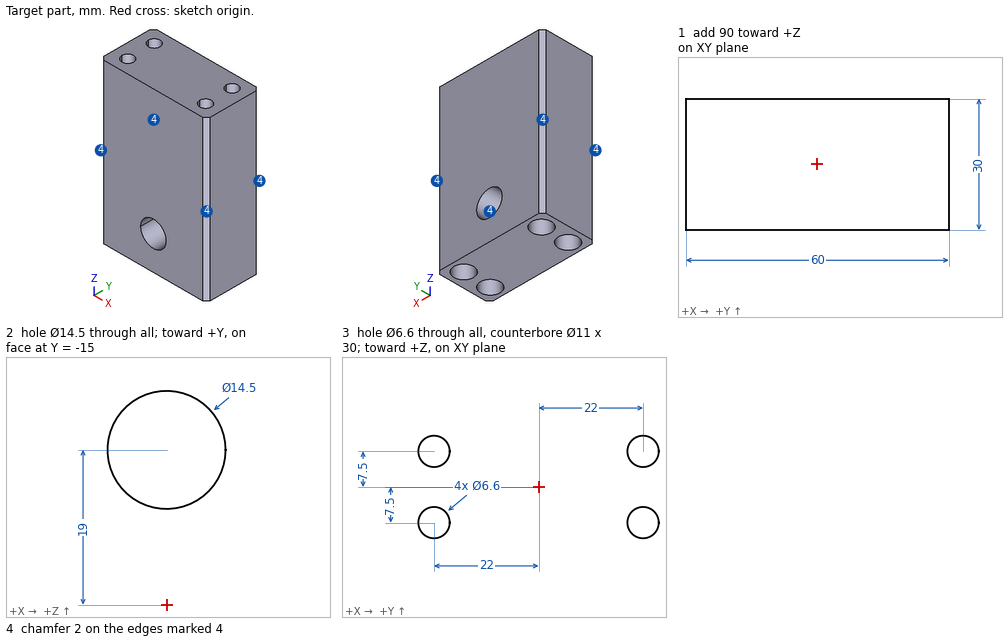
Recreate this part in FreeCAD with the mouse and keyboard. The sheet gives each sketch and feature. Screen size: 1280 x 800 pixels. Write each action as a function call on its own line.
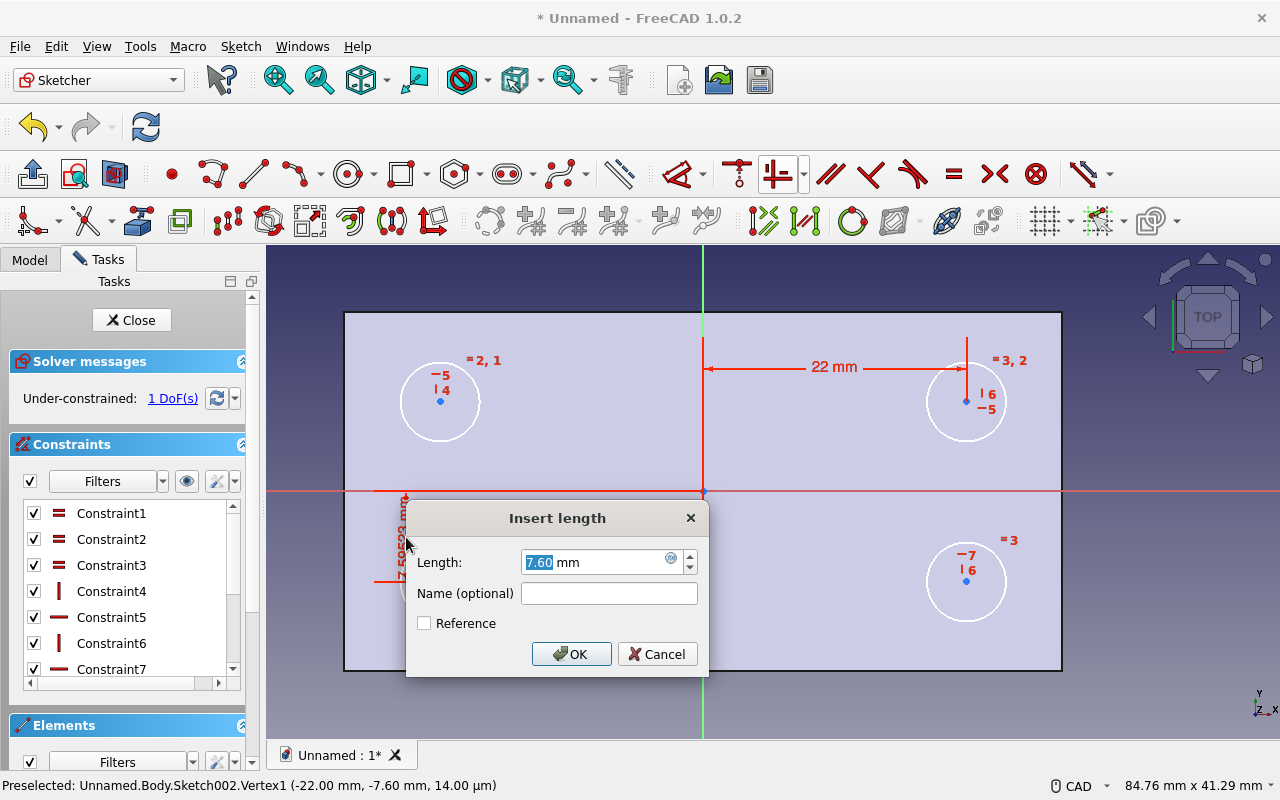
text(7.5)
key(Return)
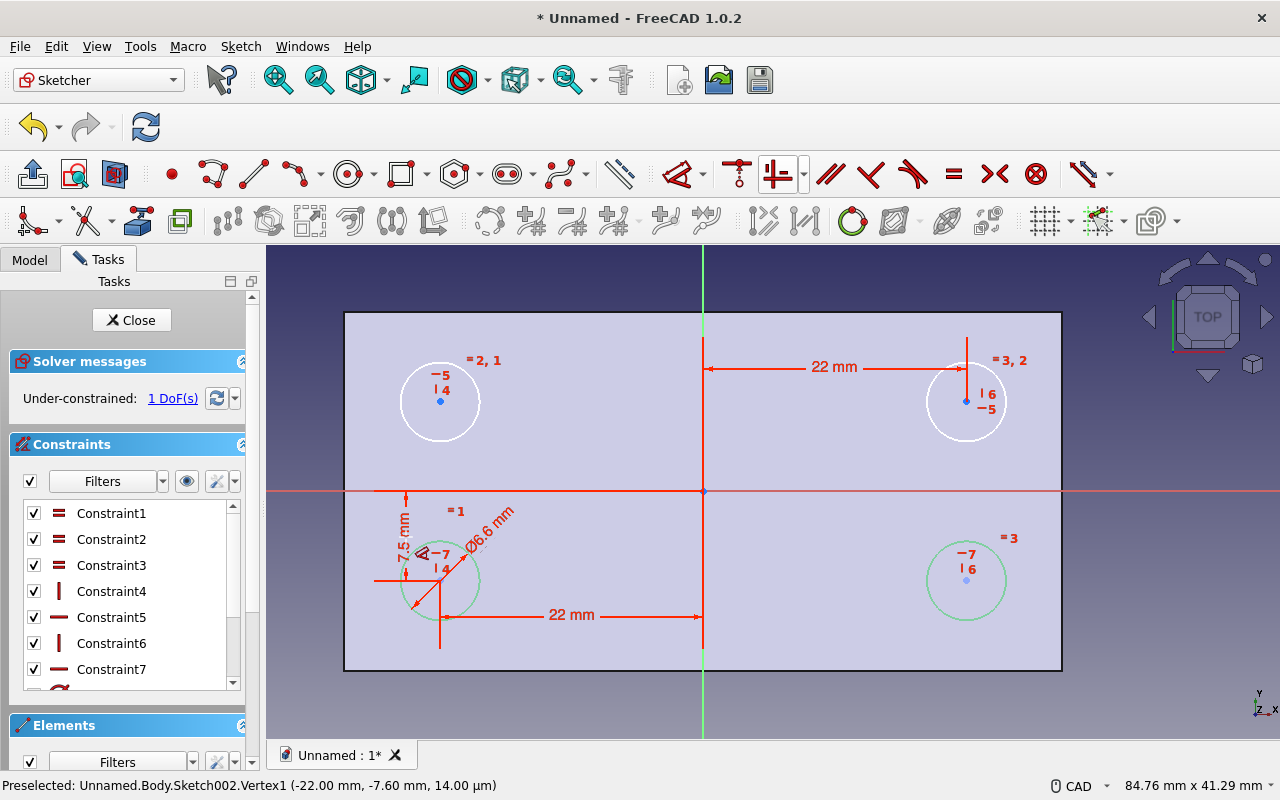
click(440, 402)
click(406, 447)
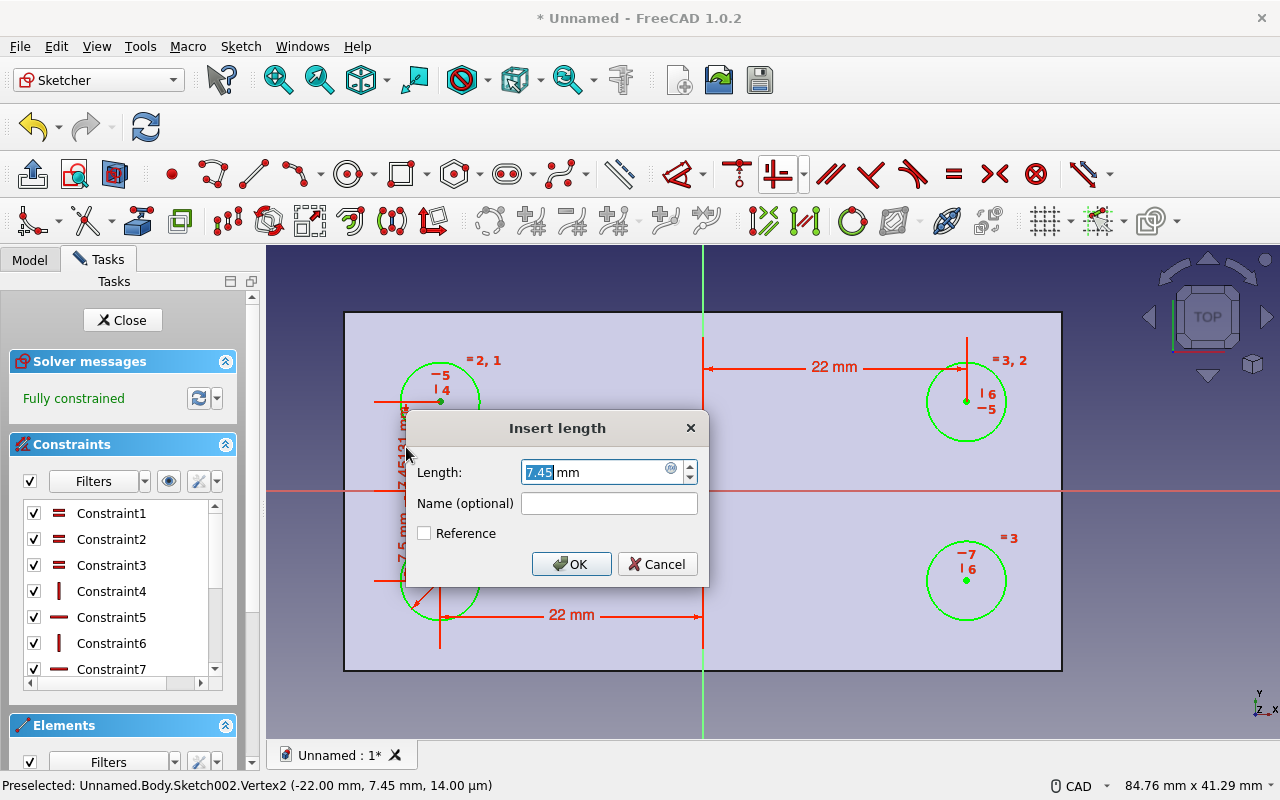
text(7.5)
key(Return)
key(Escape)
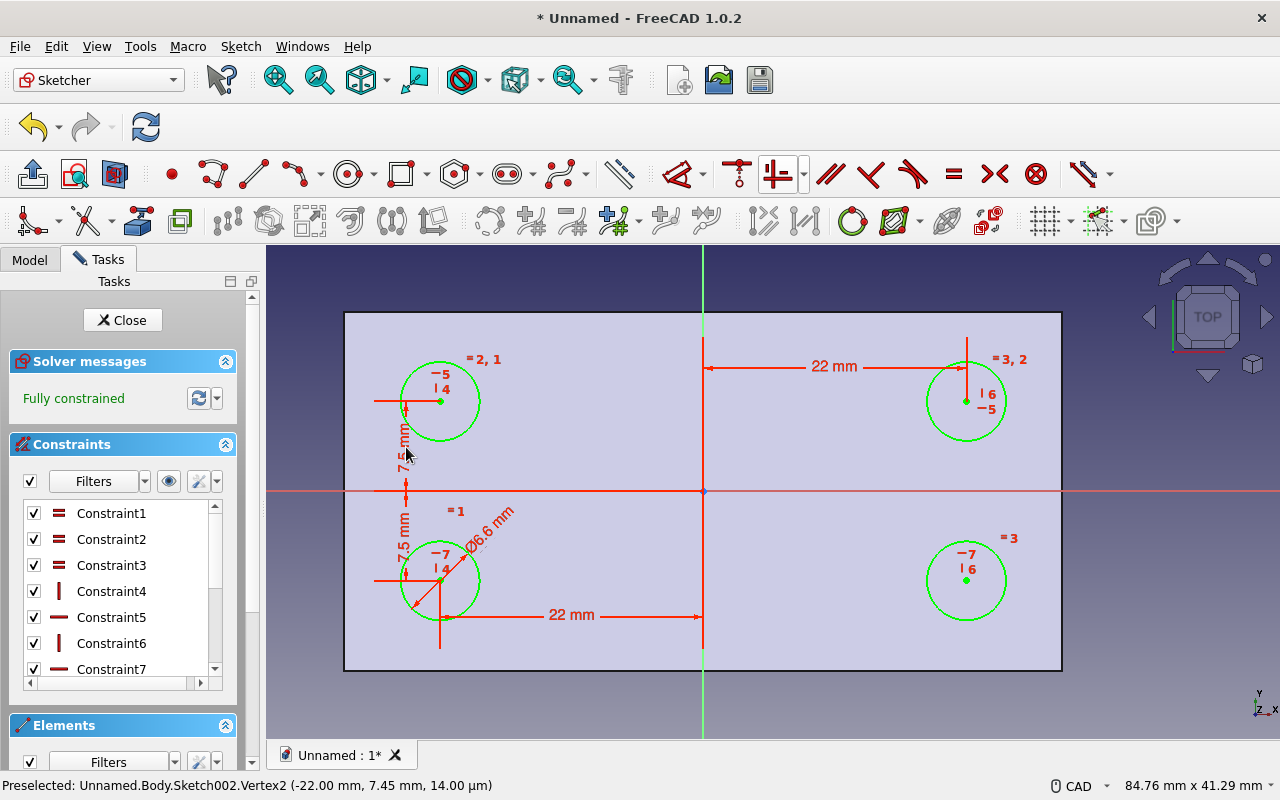
click(123, 320)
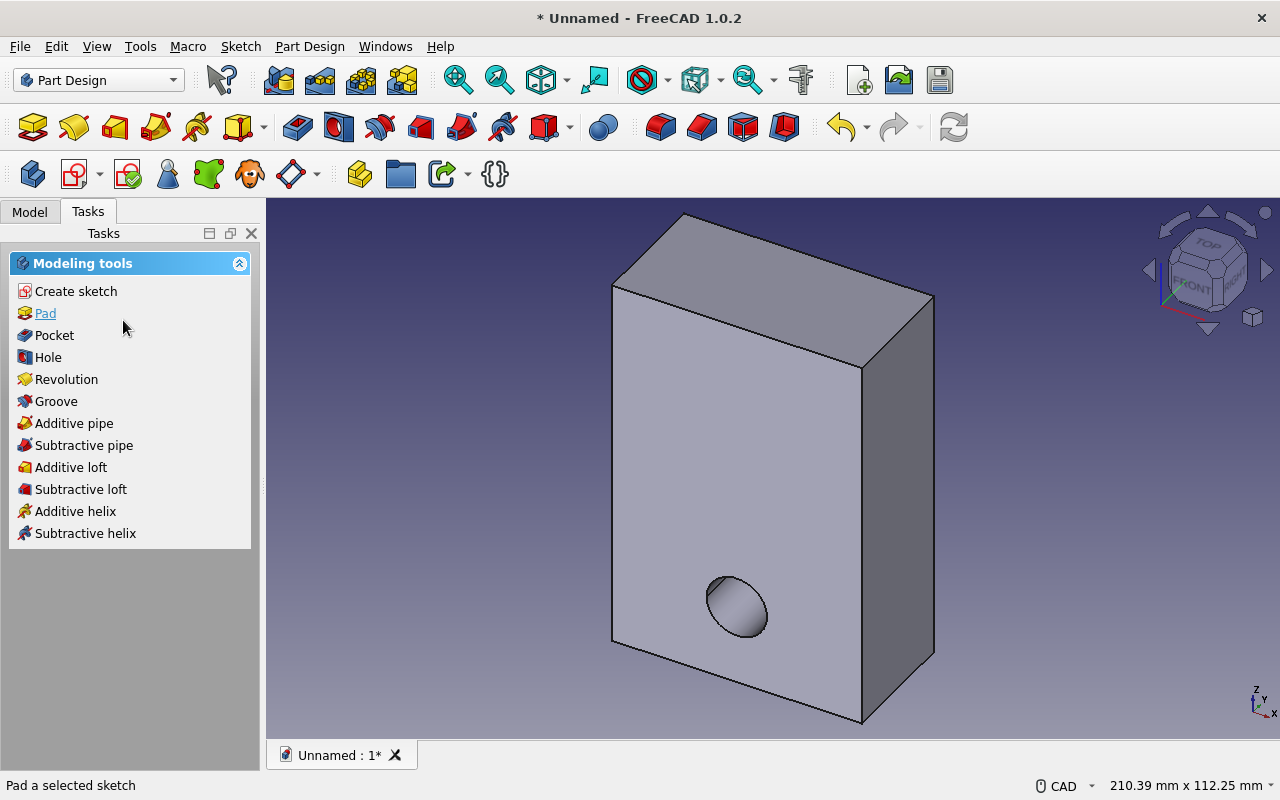
click(339, 128)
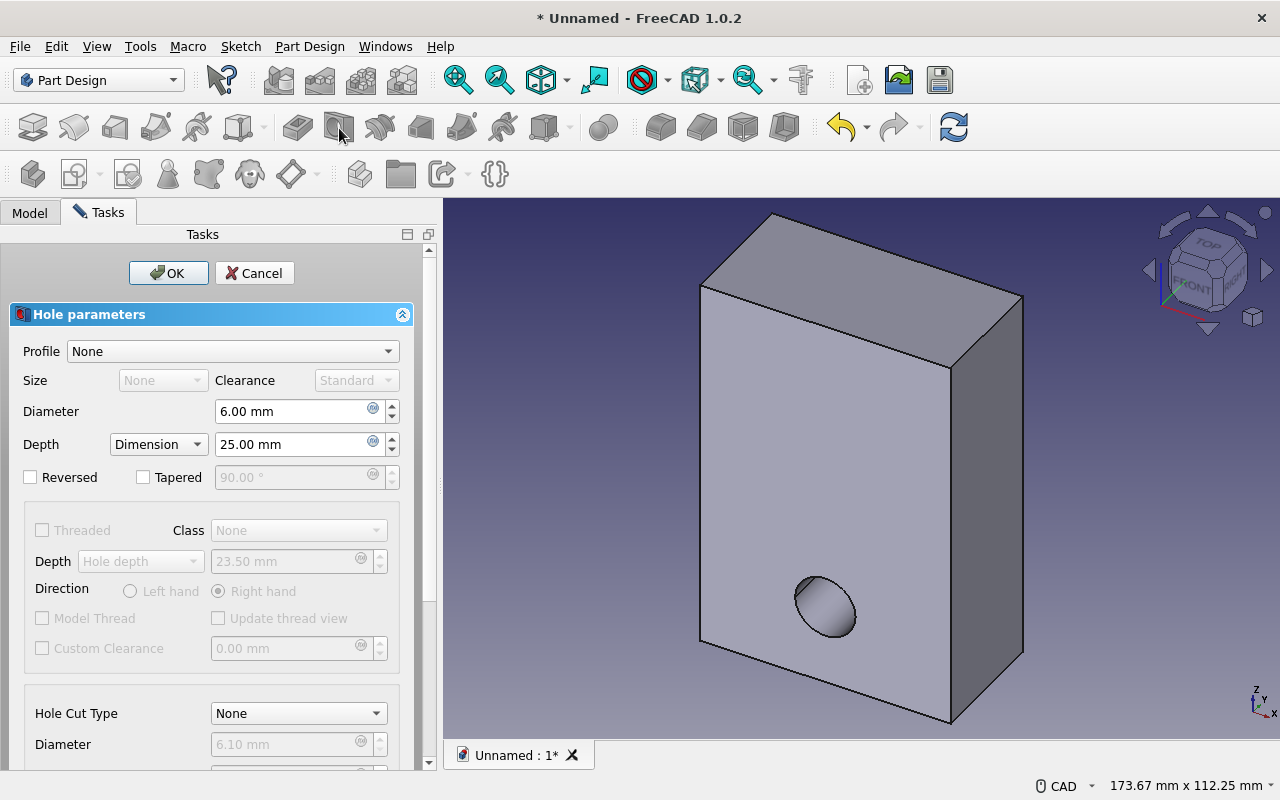
triple_click(300, 412)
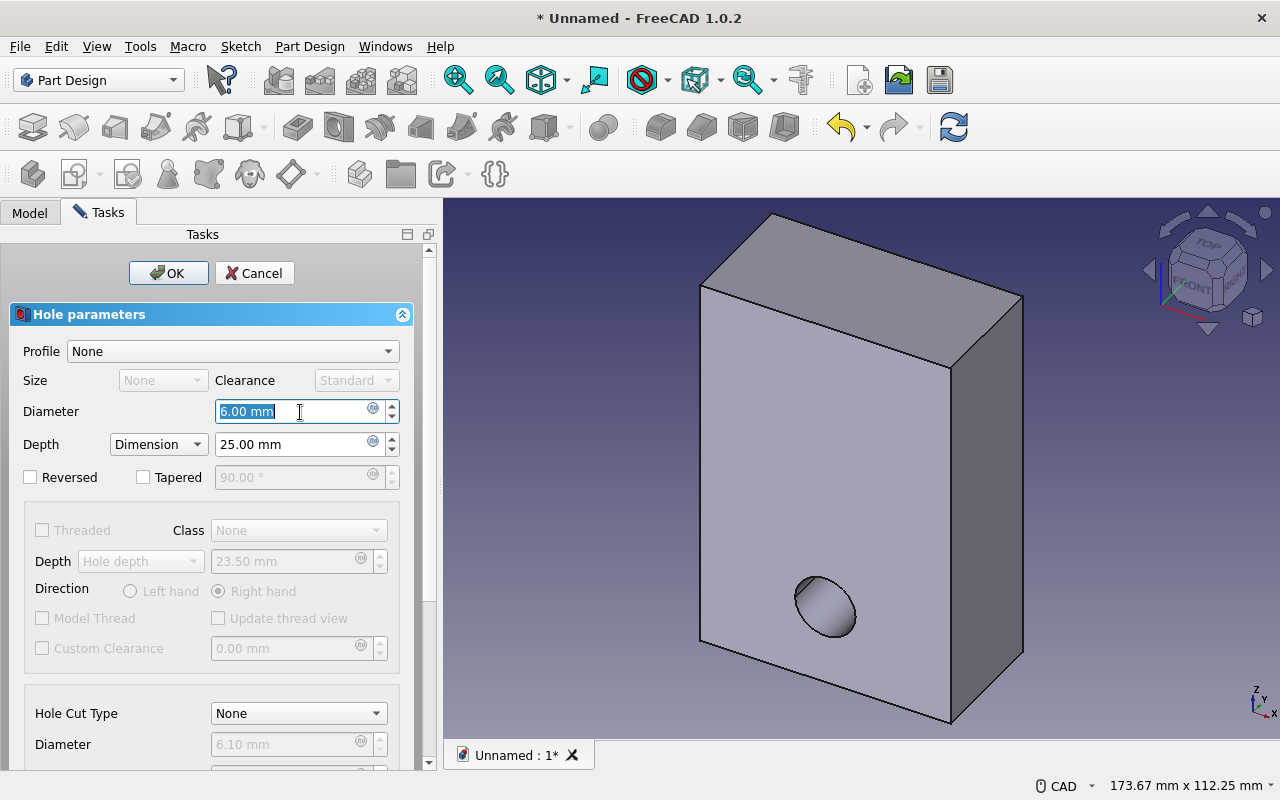
text(6.6)
key(Tab)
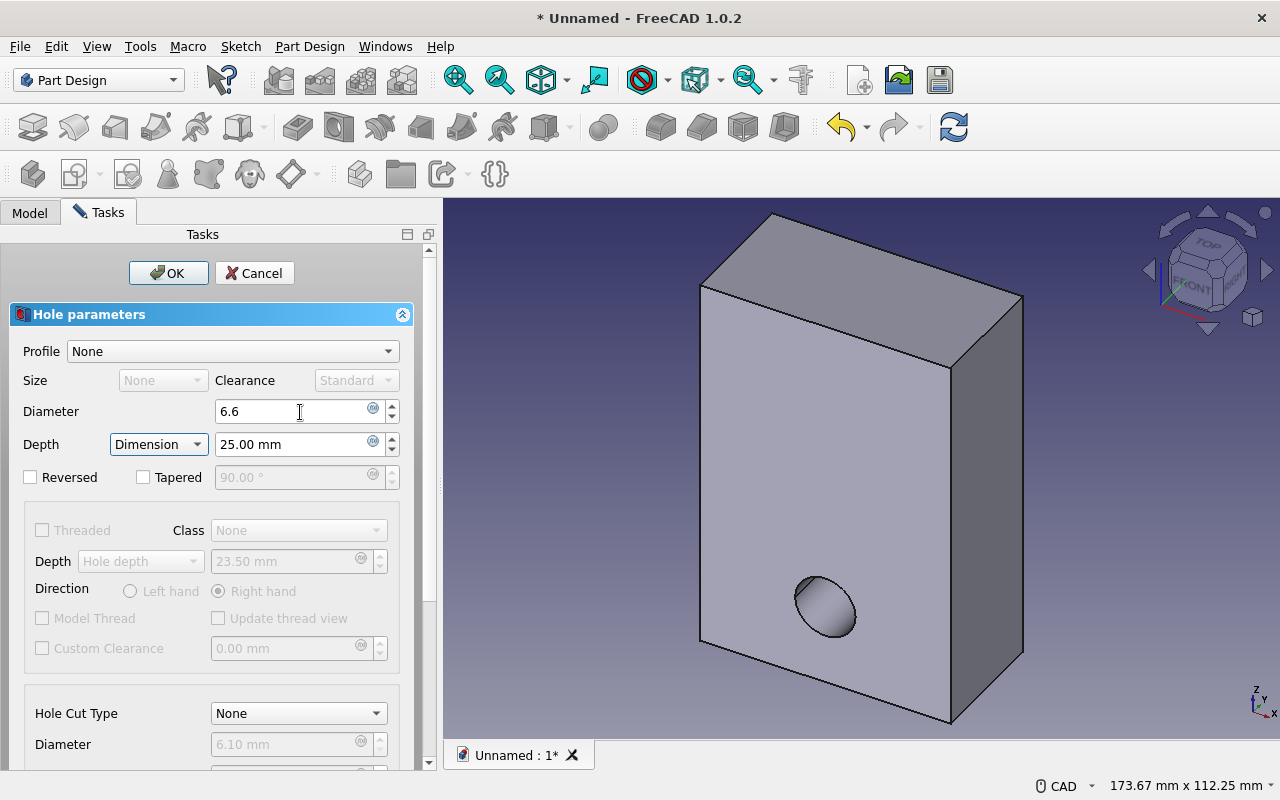
click(160, 444)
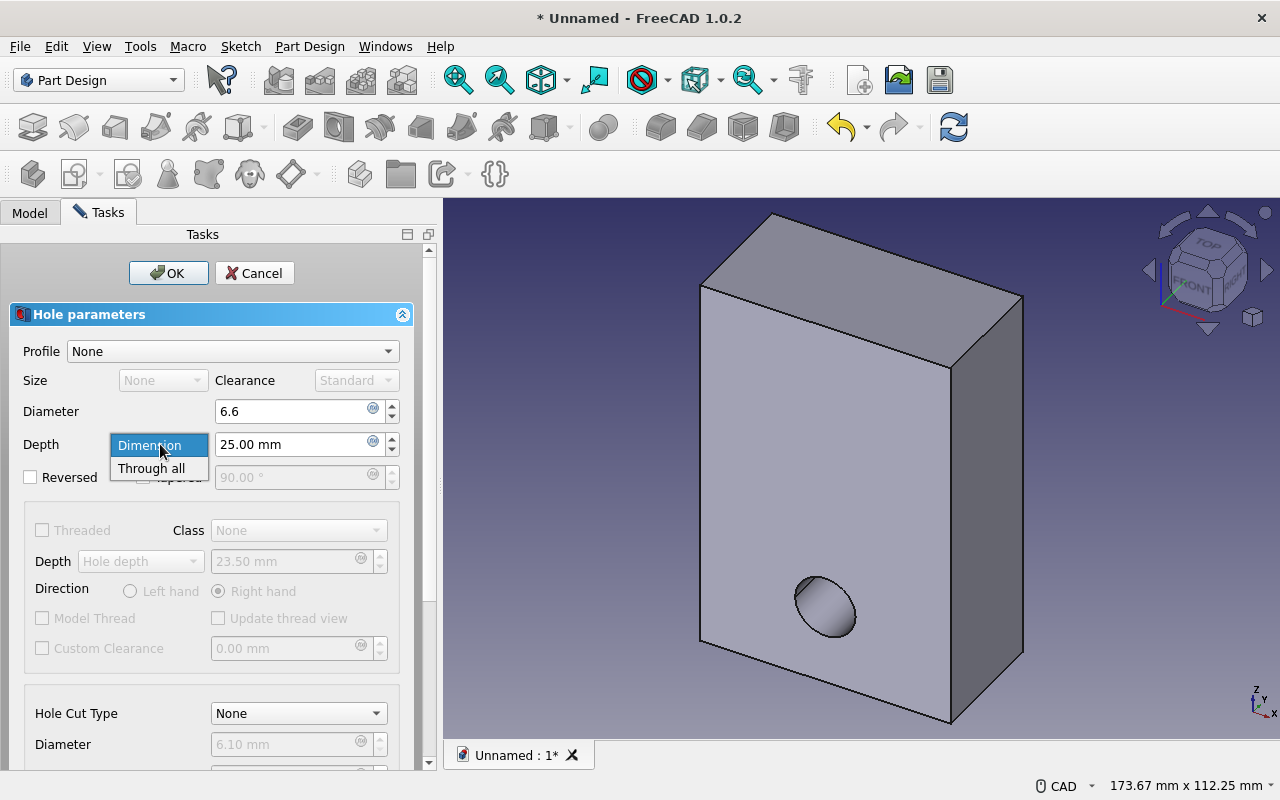
click(158, 468)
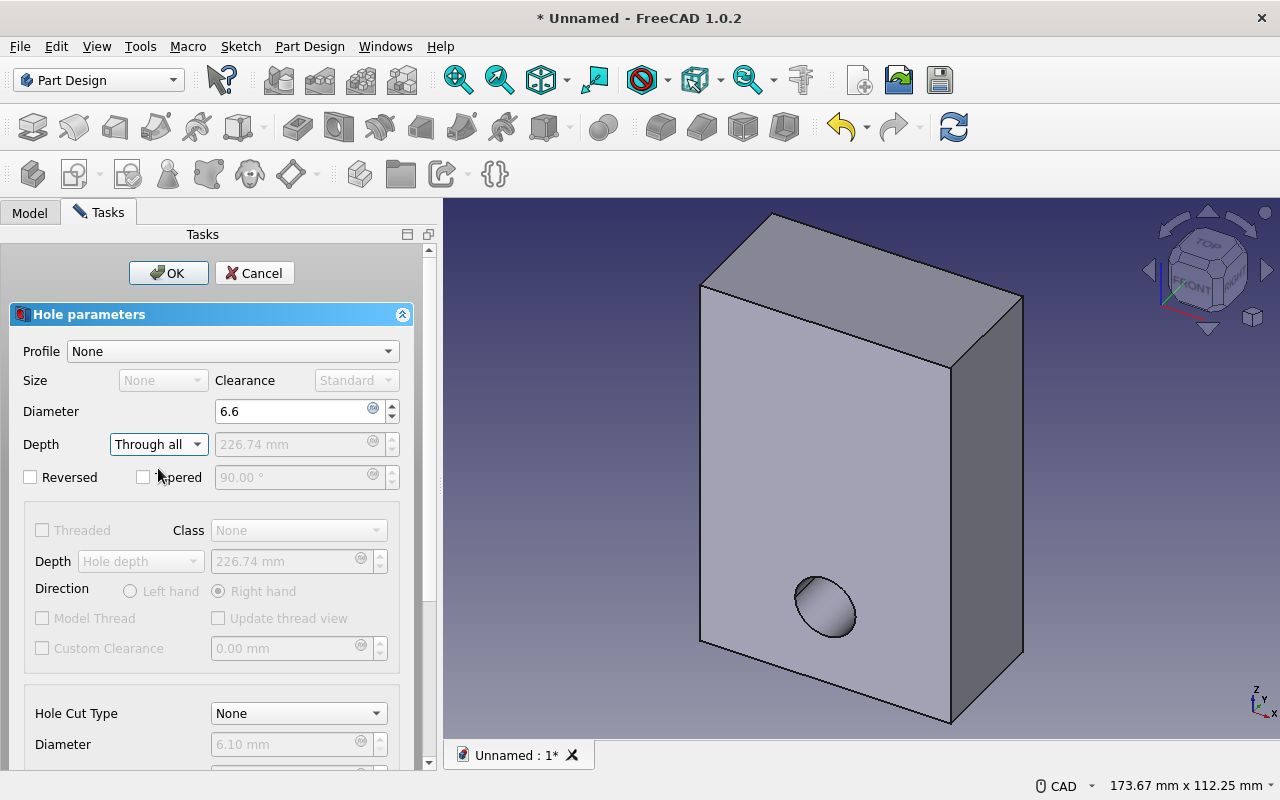
click(31, 477)